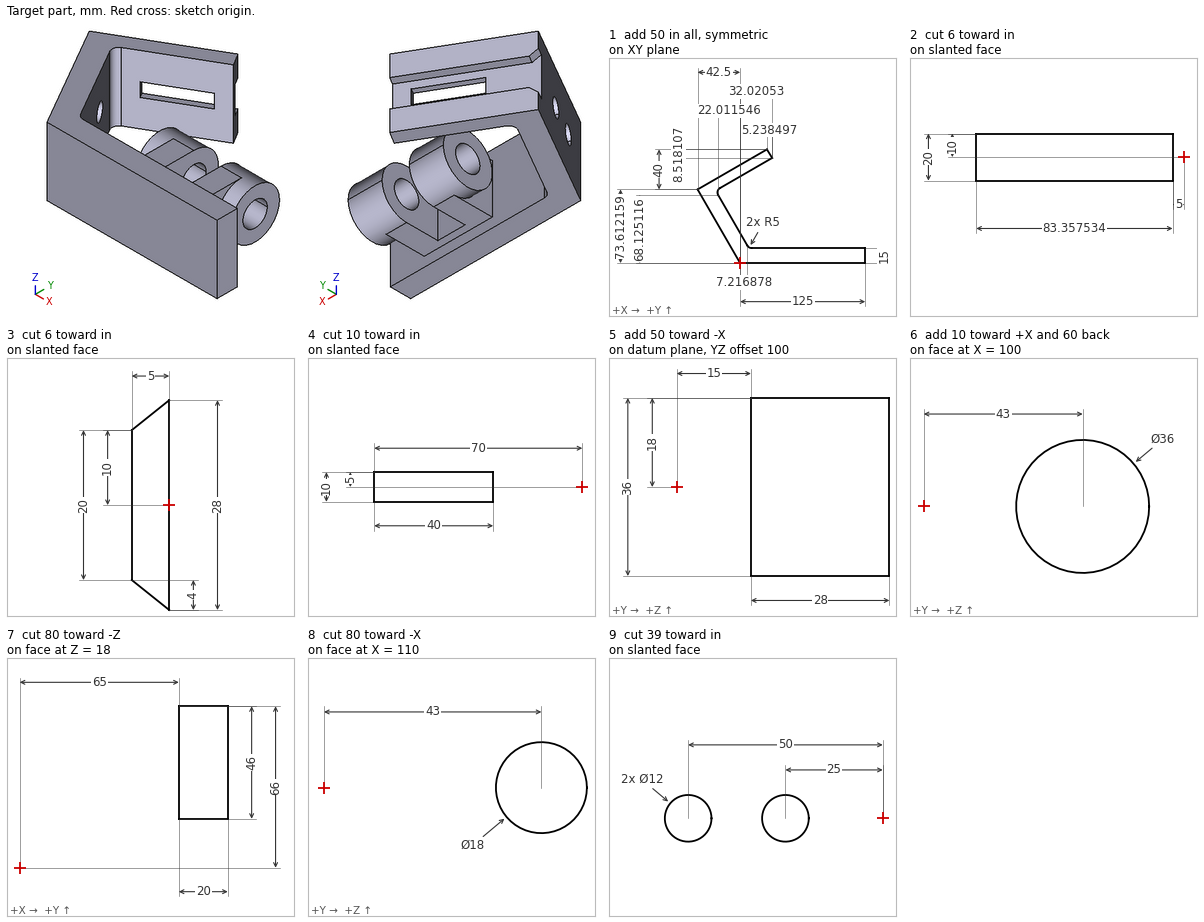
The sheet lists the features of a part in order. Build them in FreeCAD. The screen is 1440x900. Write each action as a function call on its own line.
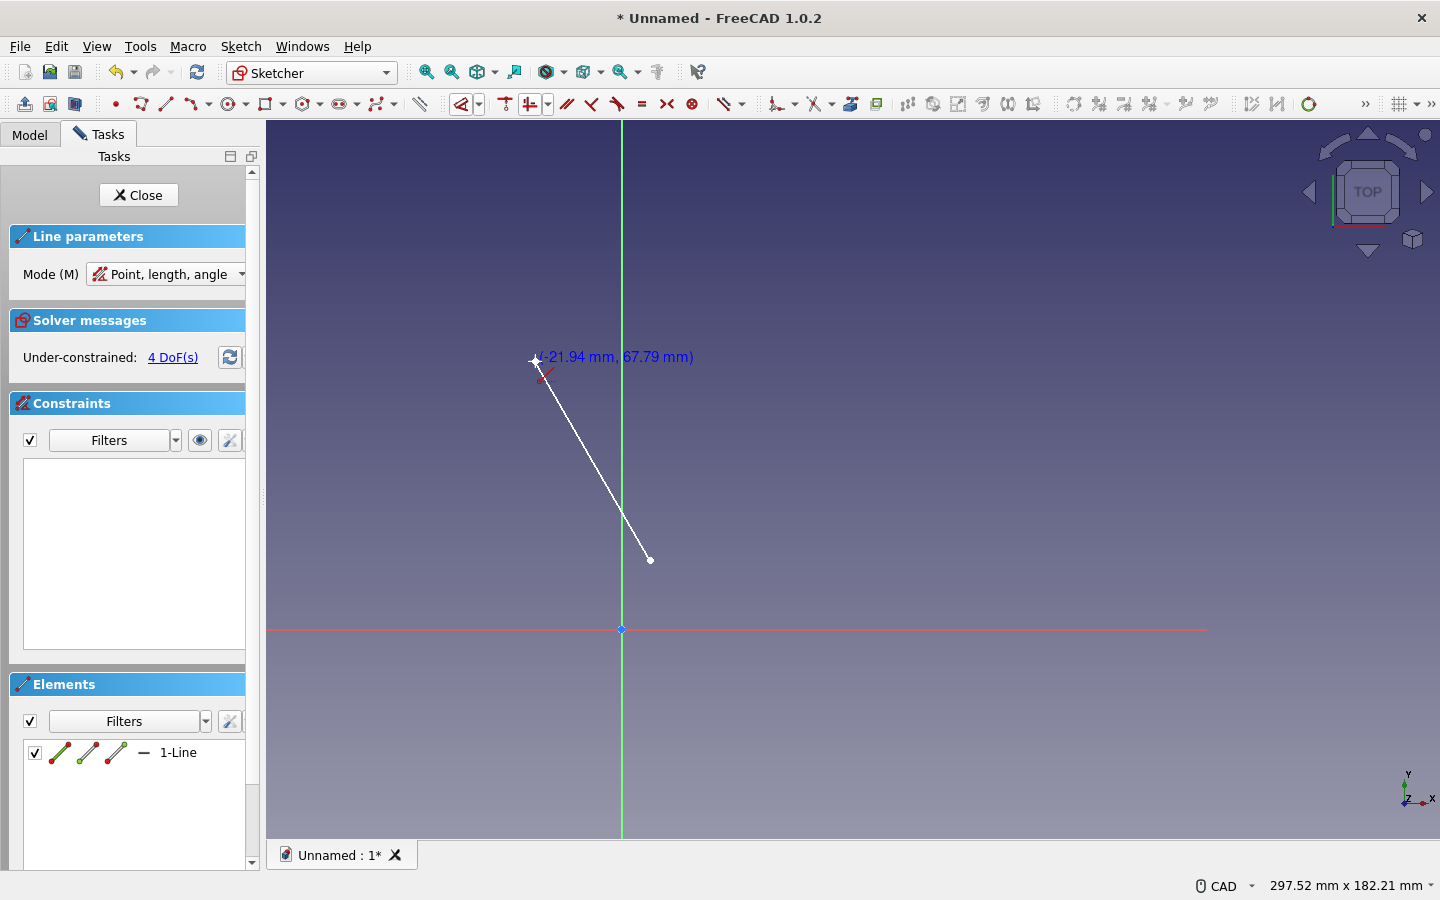
key(g)
key(m)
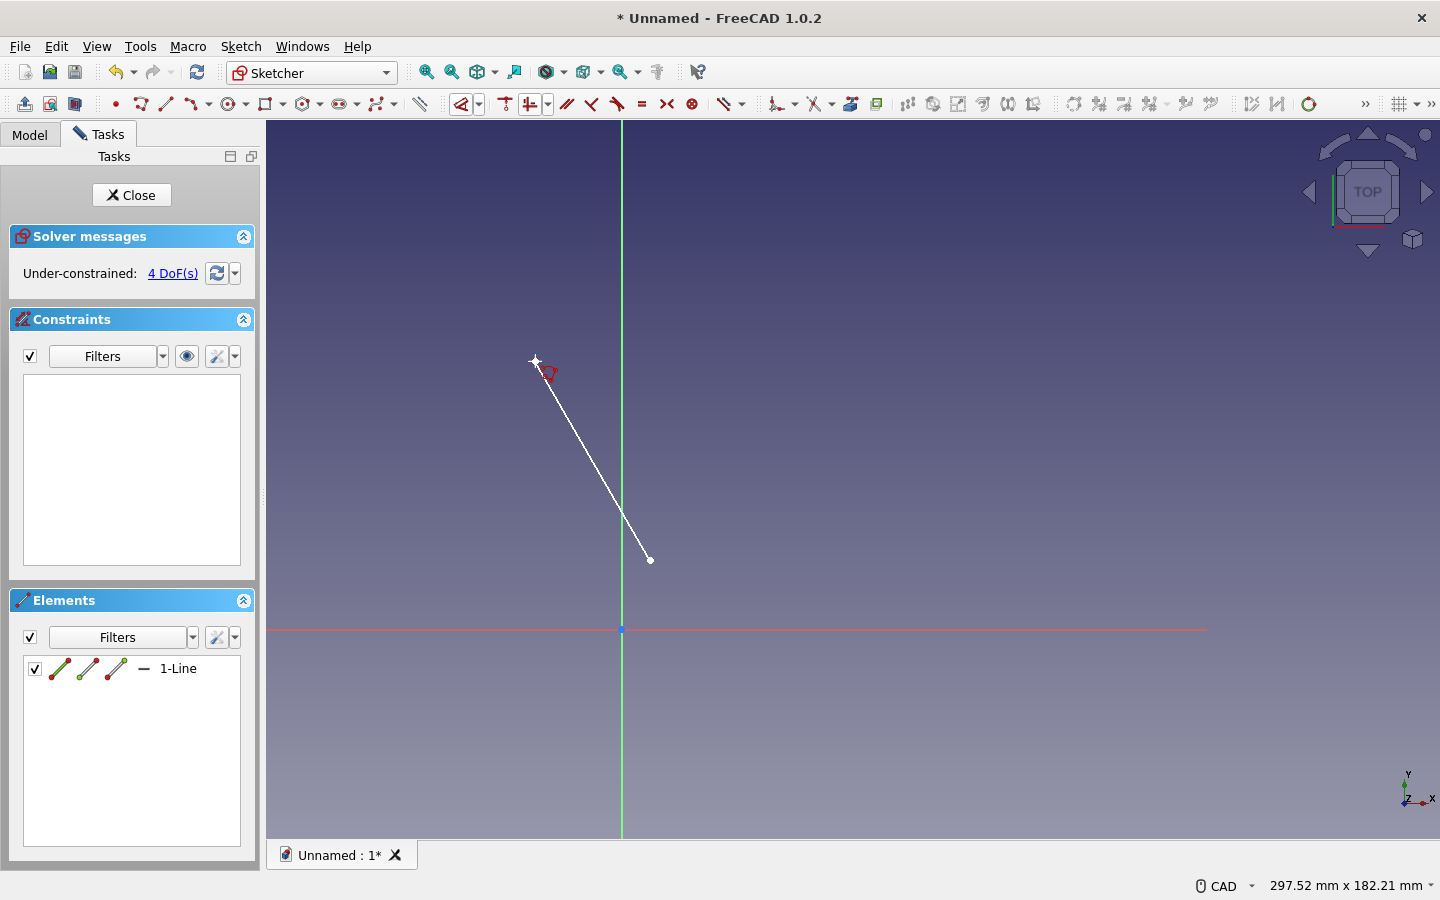
click(542, 334)
click(748, 215)
click(727, 181)
click(454, 339)
click(622, 630)
click(1115, 621)
click(1115, 570)
click(667, 570)
right_click(667, 570)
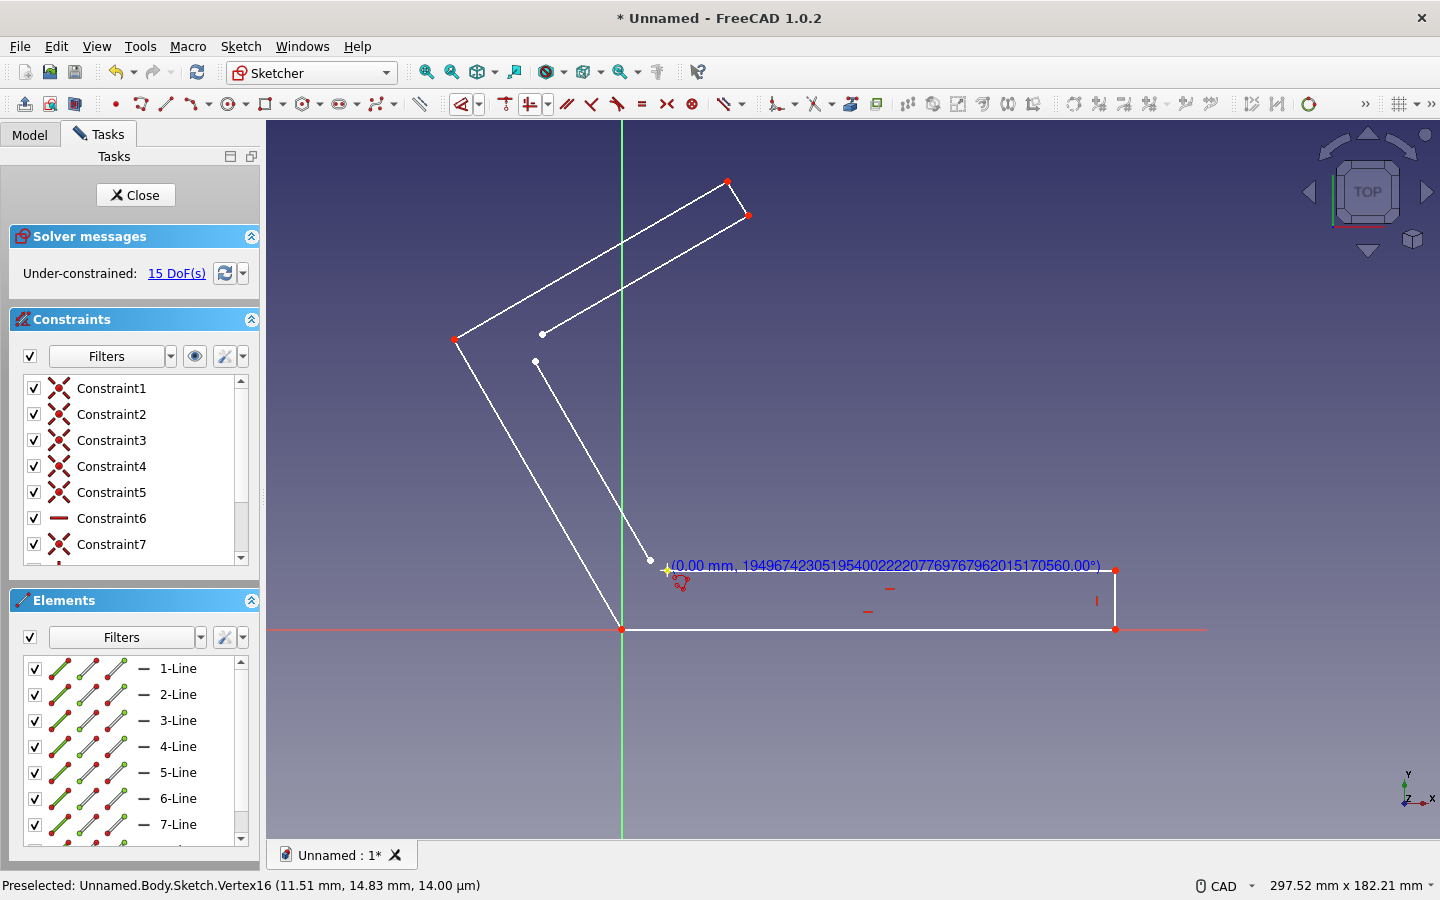
click(190, 104)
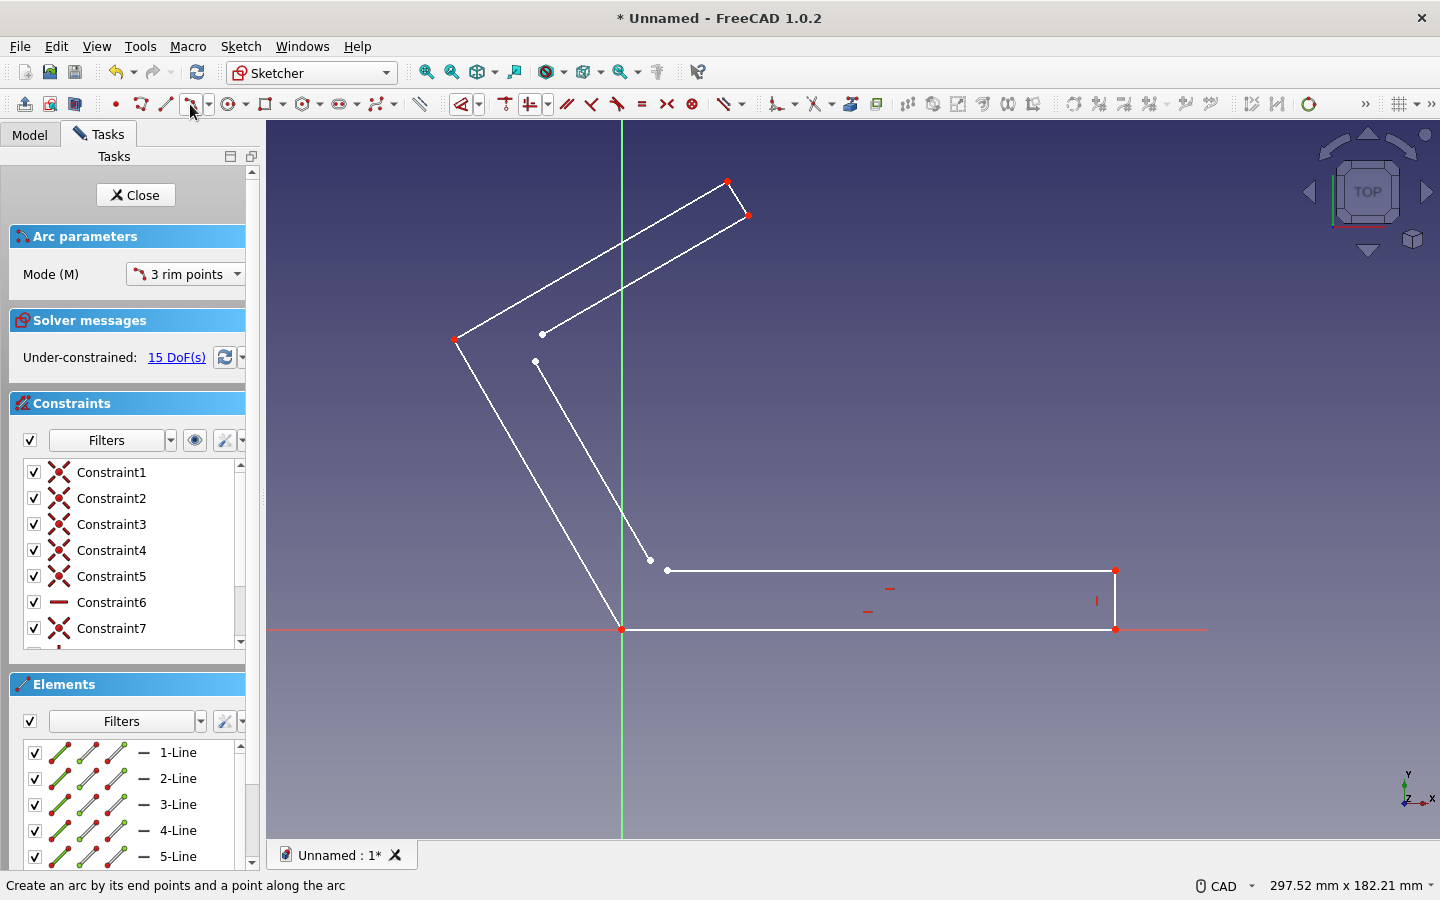
click(535, 362)
click(542, 335)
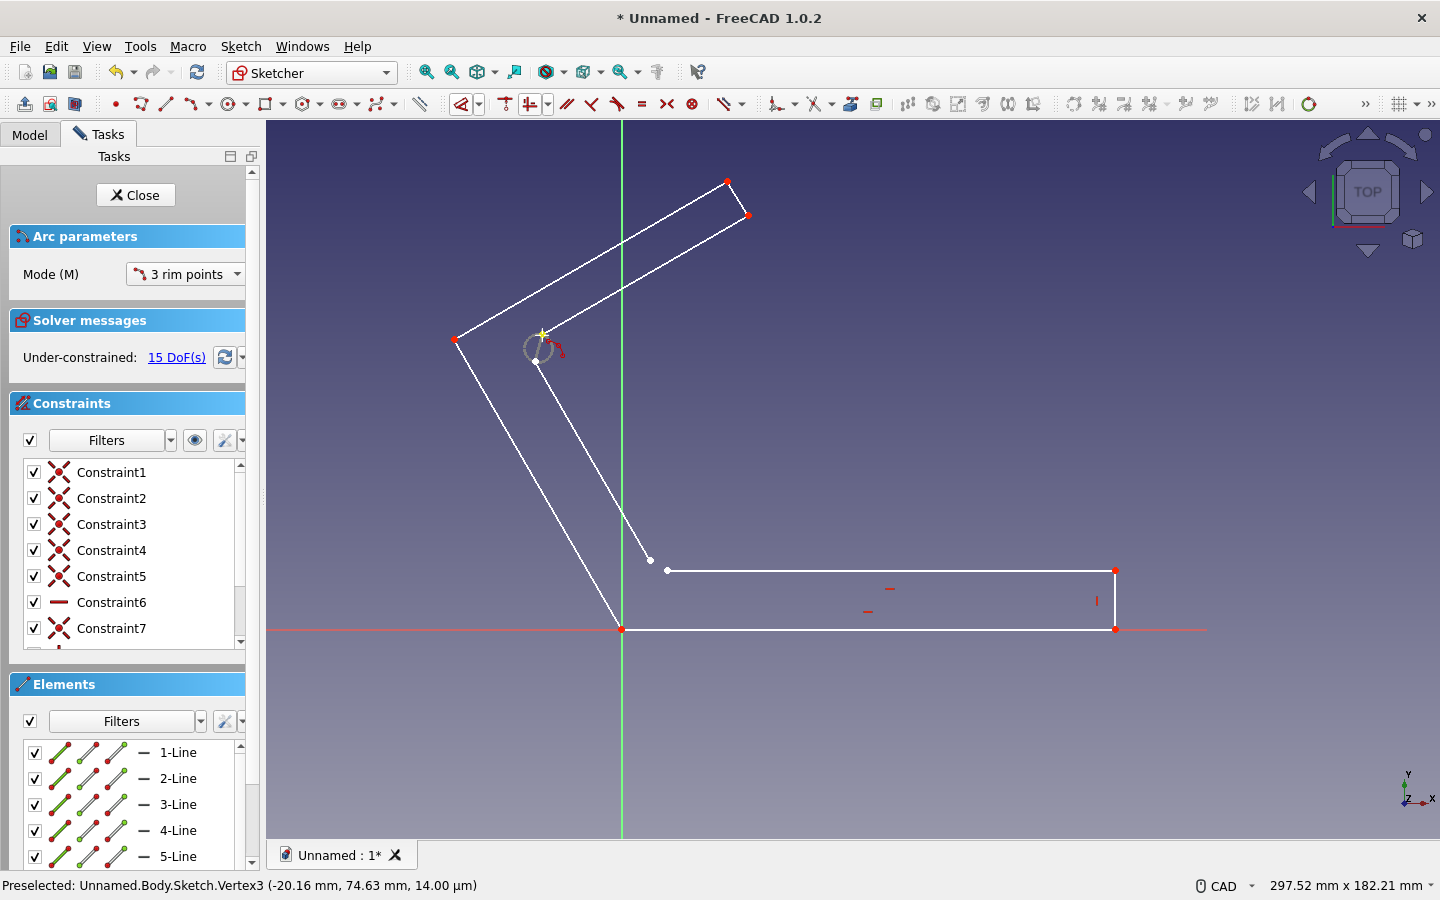
scroll(533, 346, up, 6)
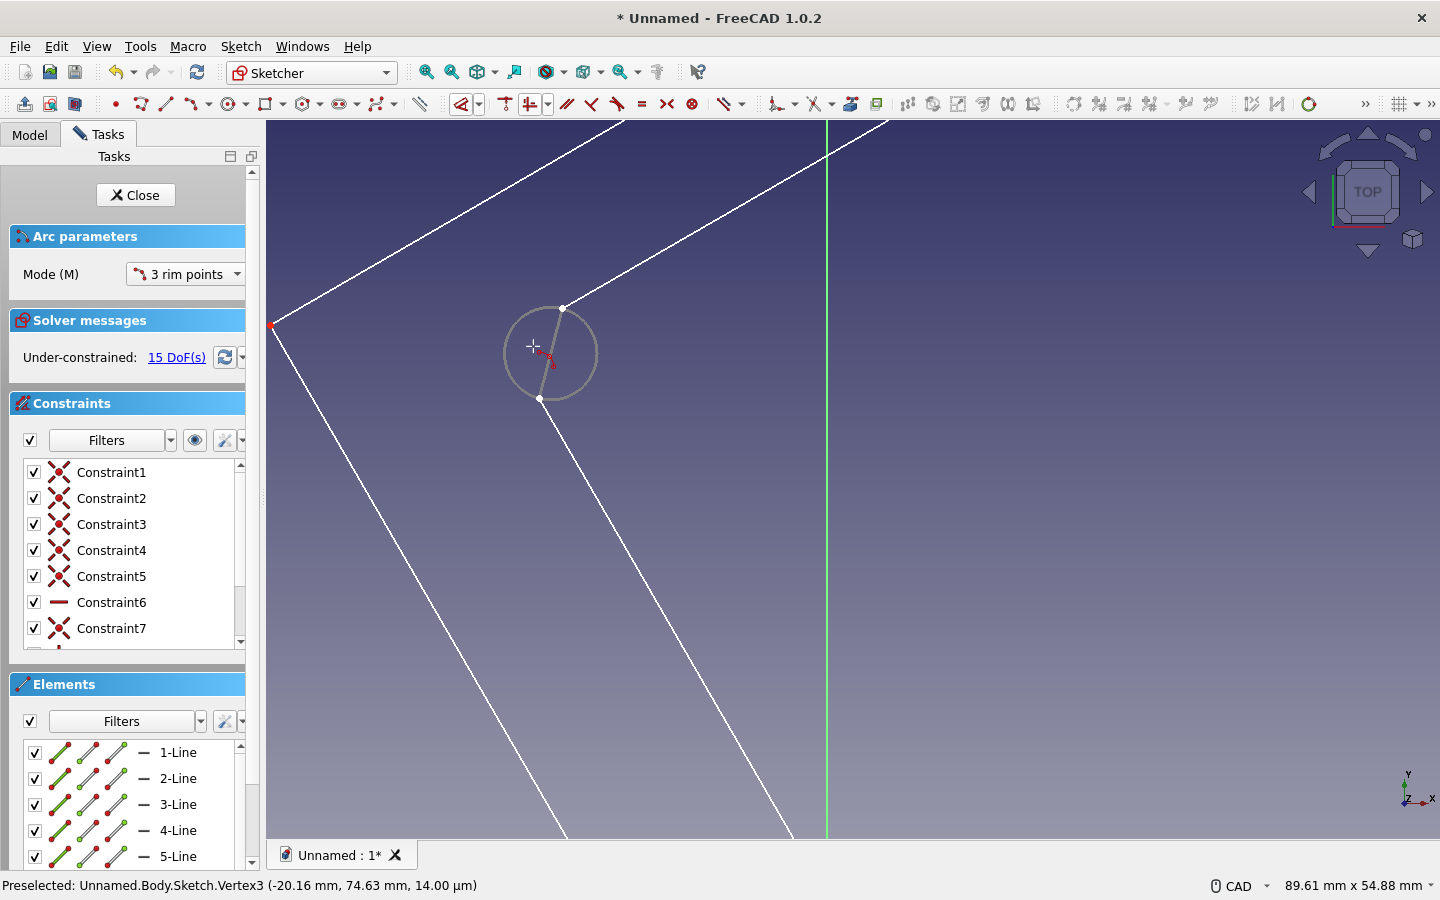
click(532, 344)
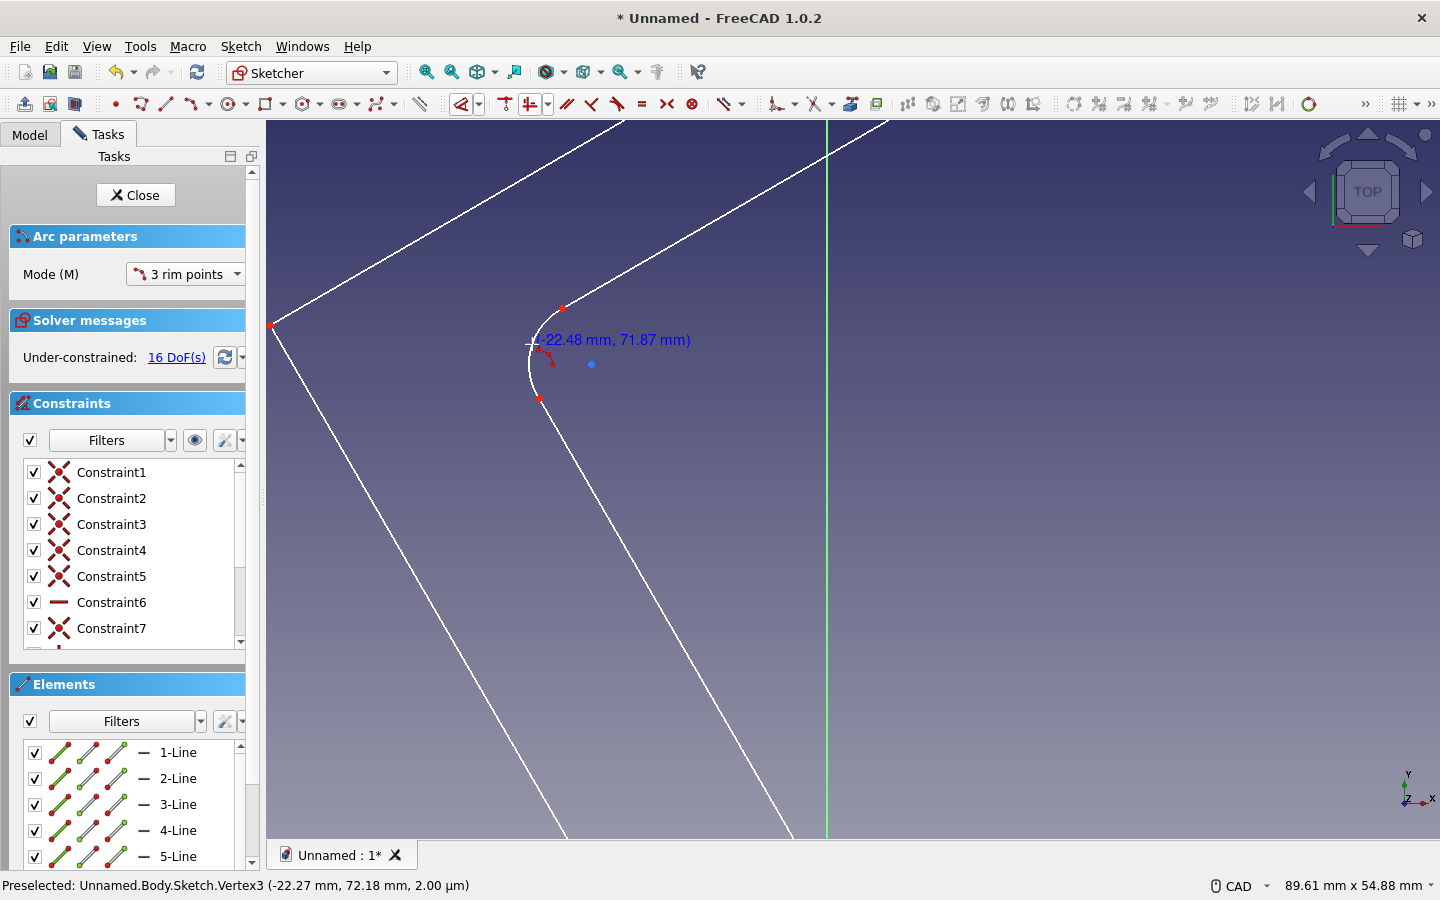
scroll(533, 452, down, 6)